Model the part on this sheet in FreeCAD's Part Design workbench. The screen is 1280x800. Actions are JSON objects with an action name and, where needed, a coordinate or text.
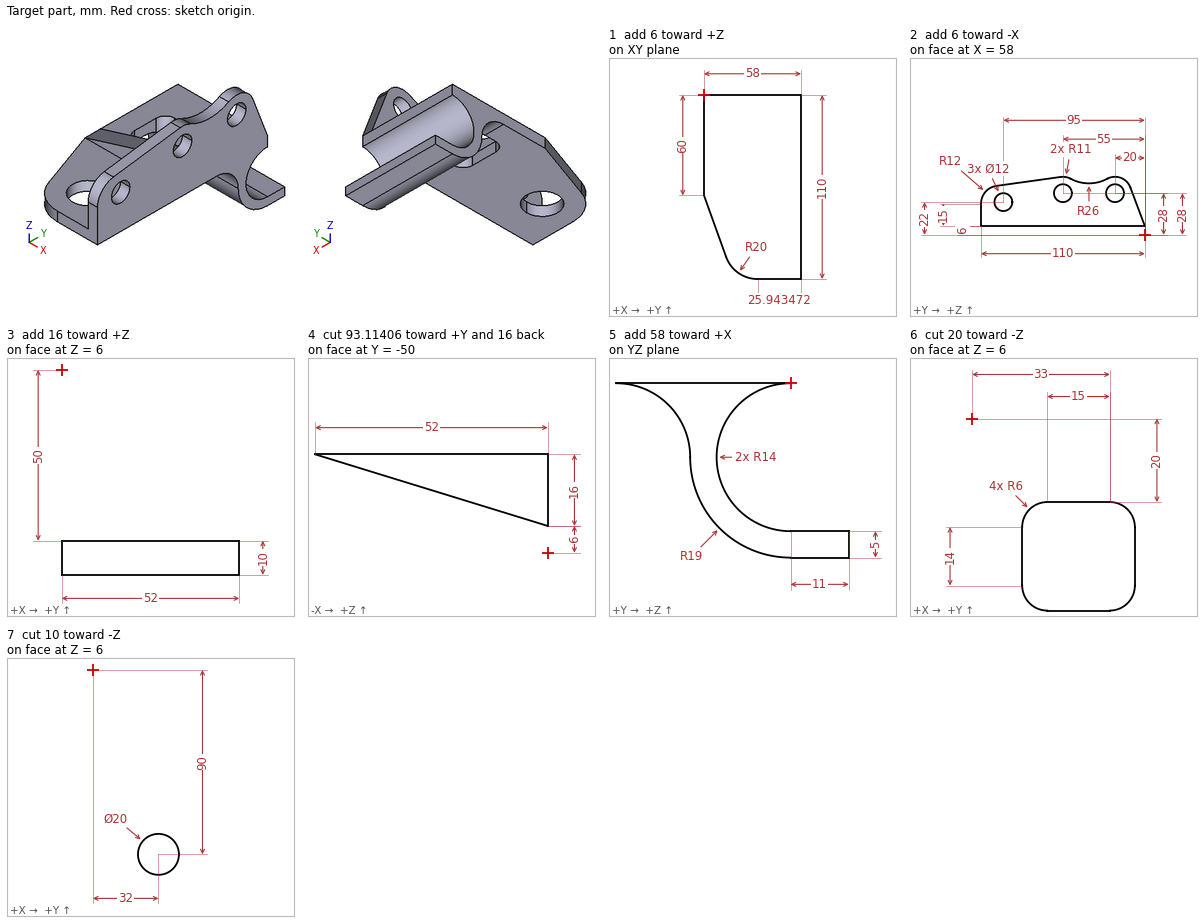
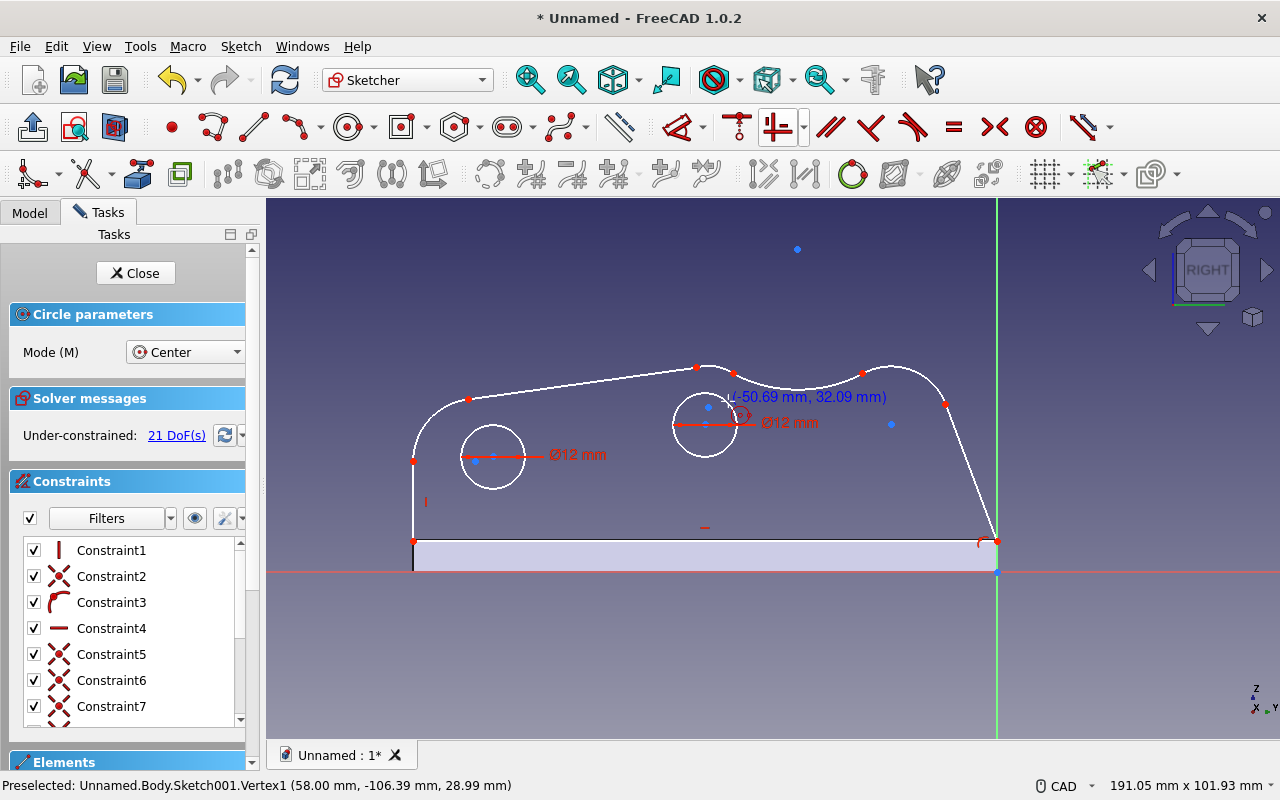
{"action": "left_click", "coordinate": [891, 424]}
{"action": "mouse_move", "coordinate": [913, 401]}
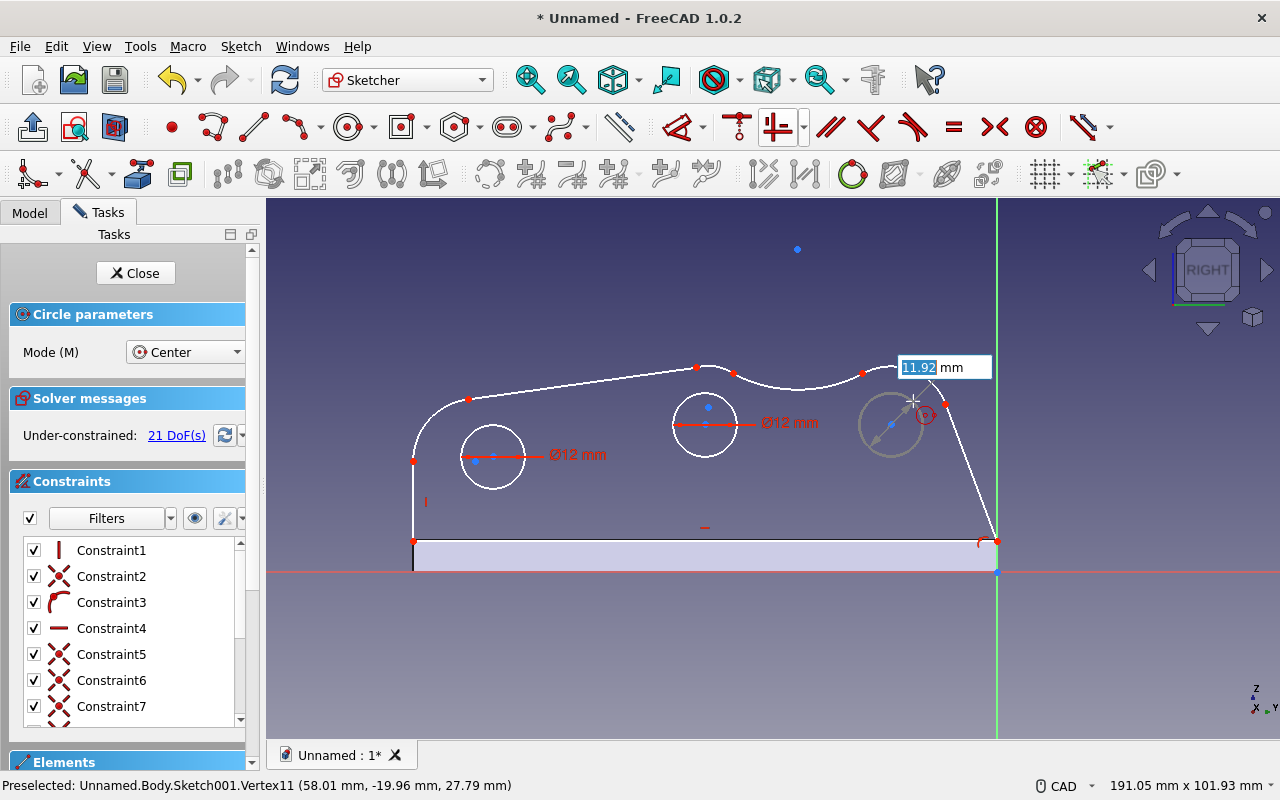
{"action": "type", "text": "12"}
{"action": "key", "text": "Return"}
{"action": "key", "text": "Escape"}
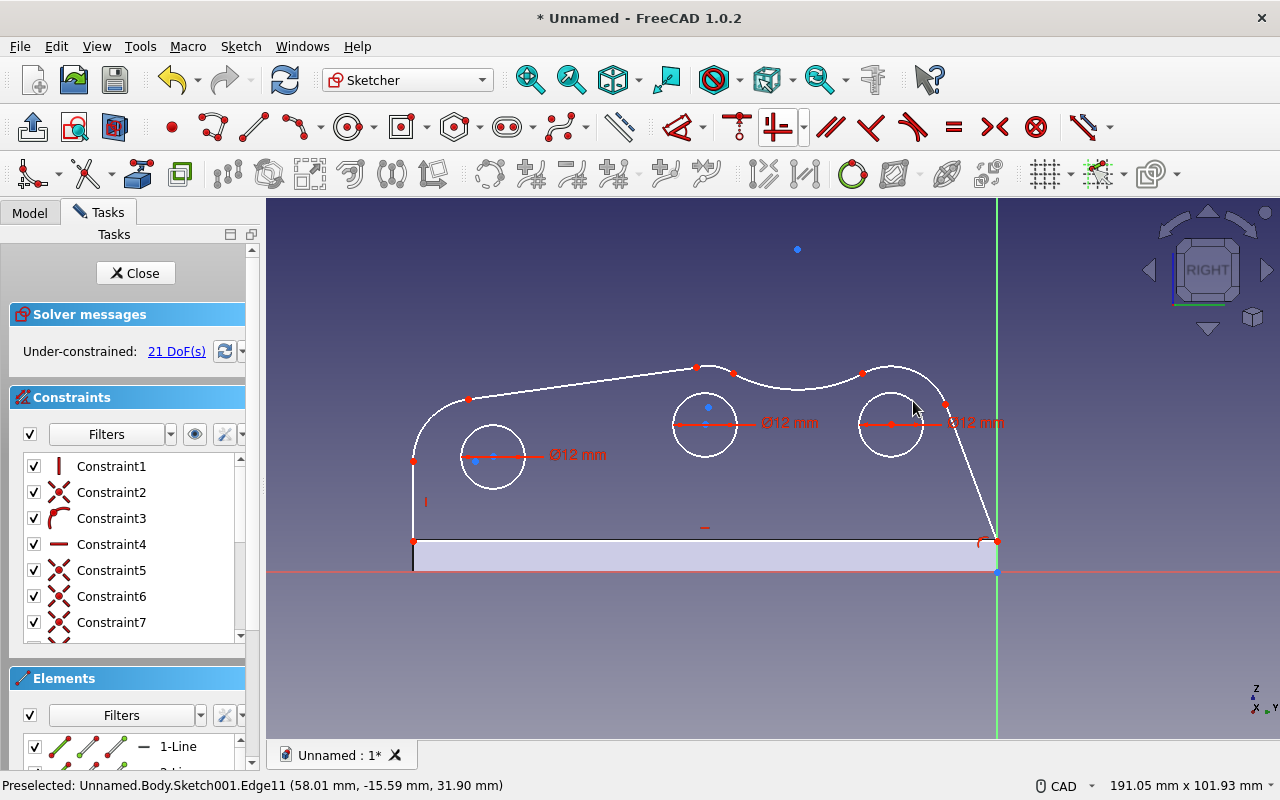
{"action": "left_click", "coordinate": [413, 486]}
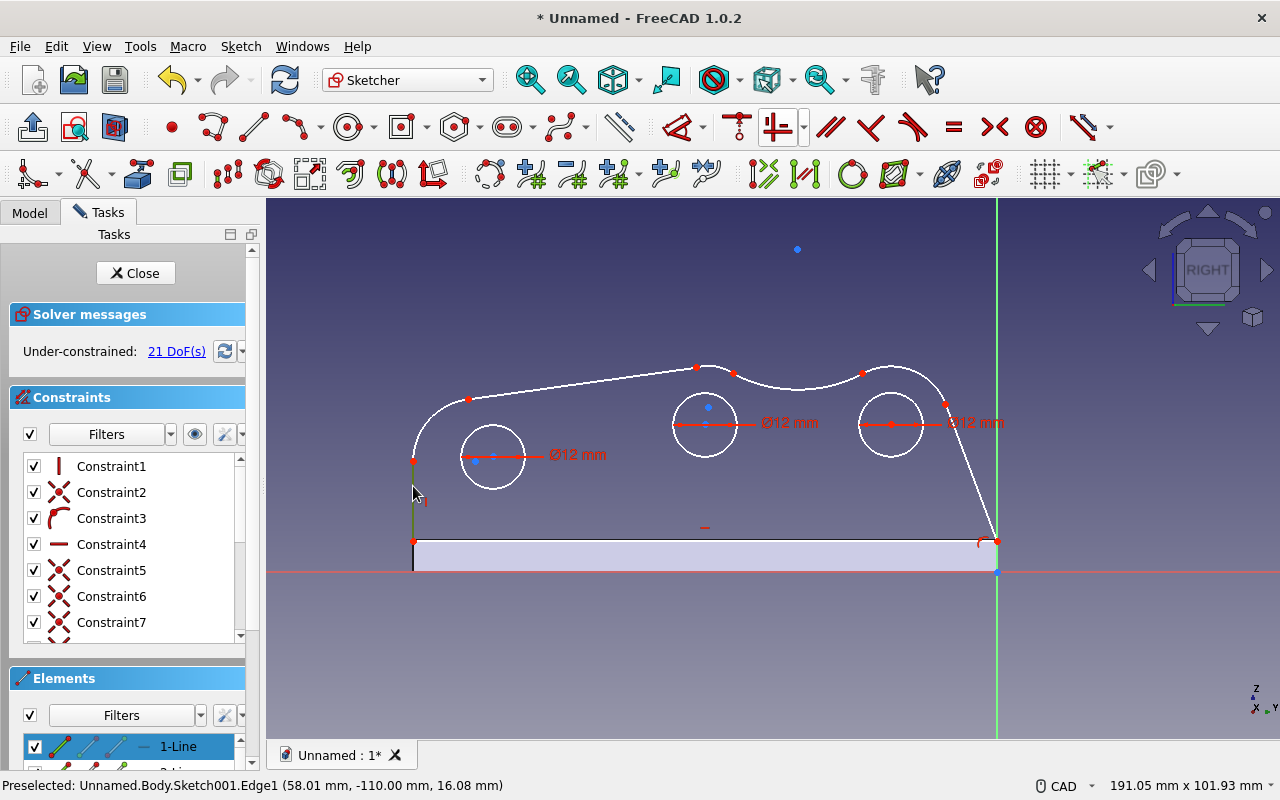
{"action": "left_click", "coordinate": [443, 408]}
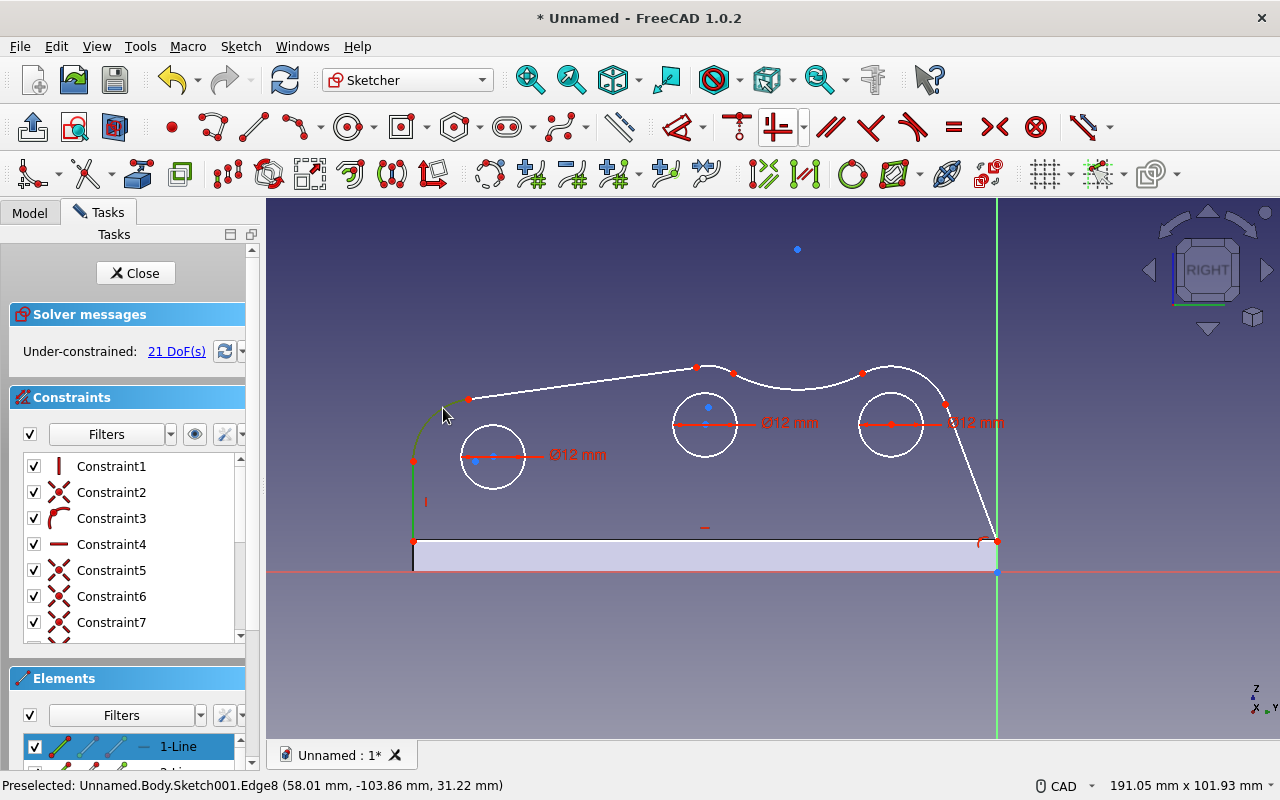
{"action": "key", "text": "t"}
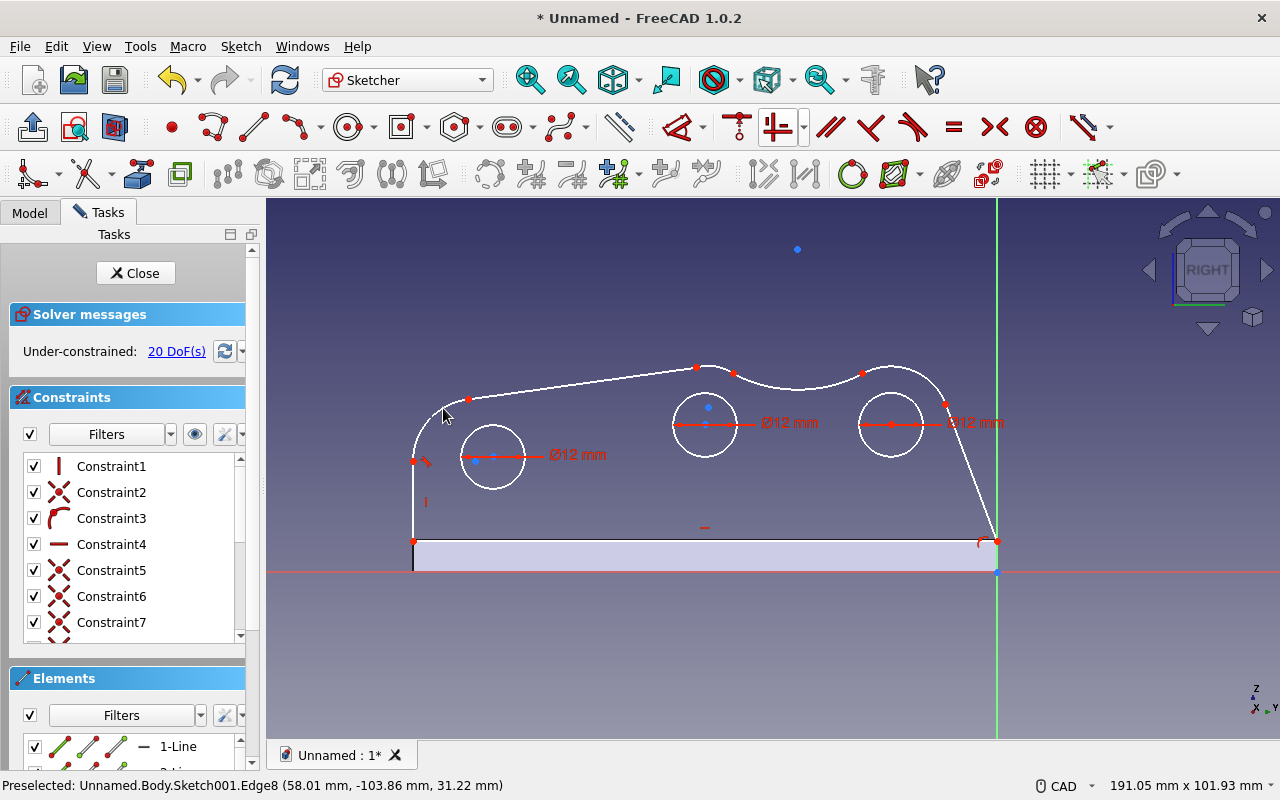
{"action": "left_click", "coordinate": [982, 500]}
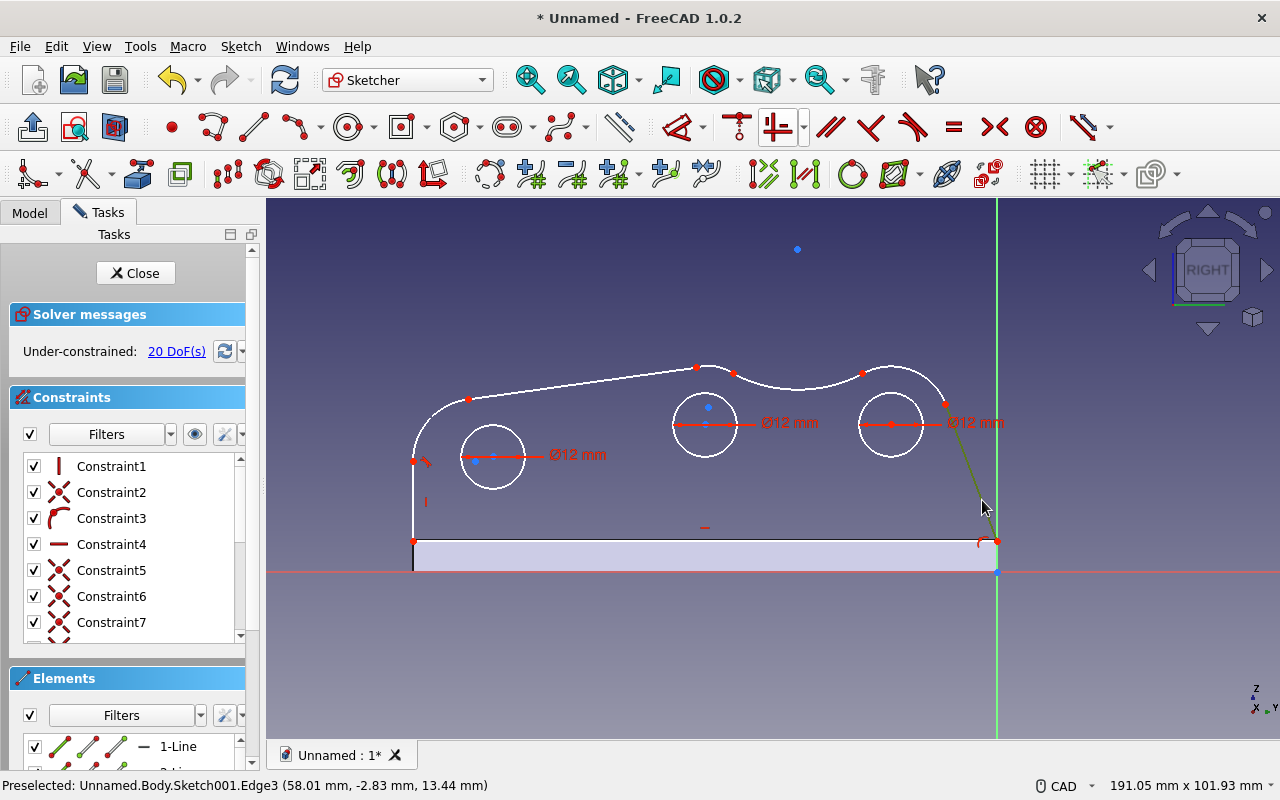
{"action": "left_click", "coordinate": [929, 380]}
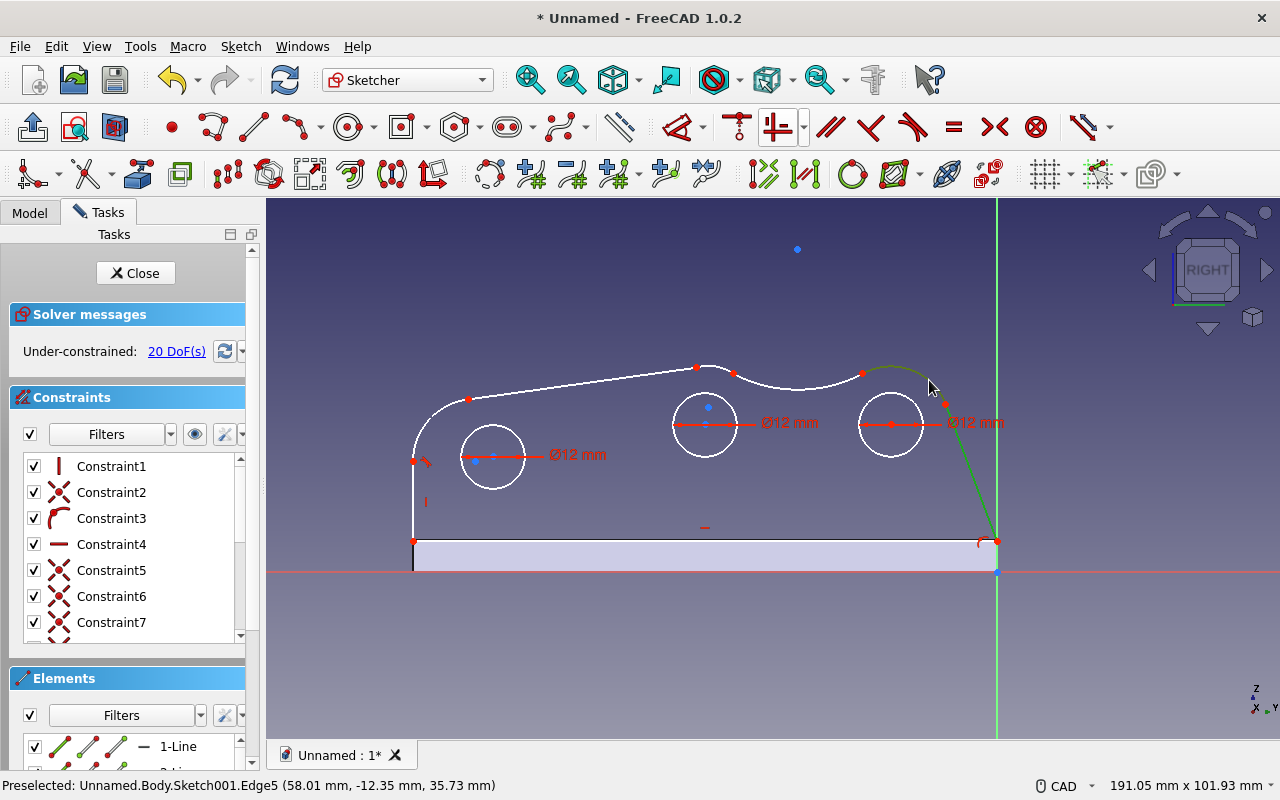
{"action": "left_click", "coordinate": [913, 128]}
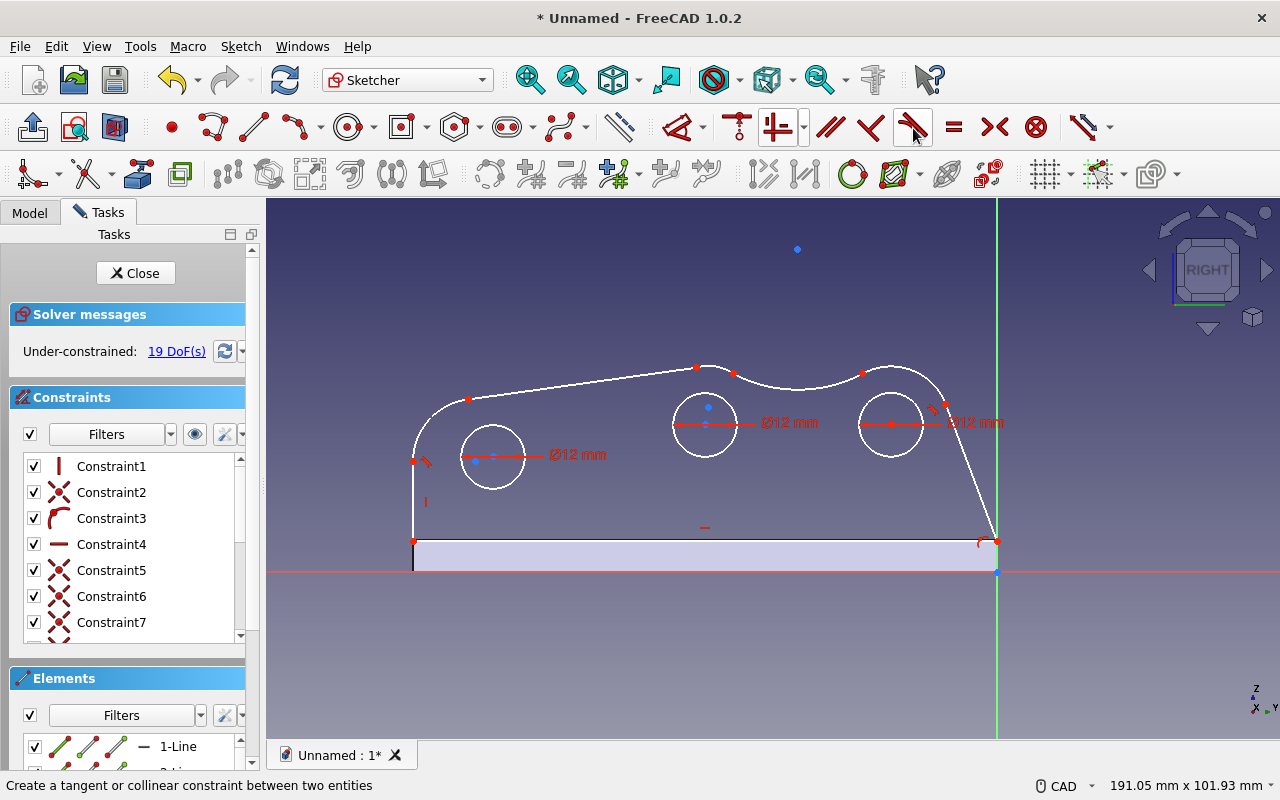
{"action": "left_click", "coordinate": [628, 377]}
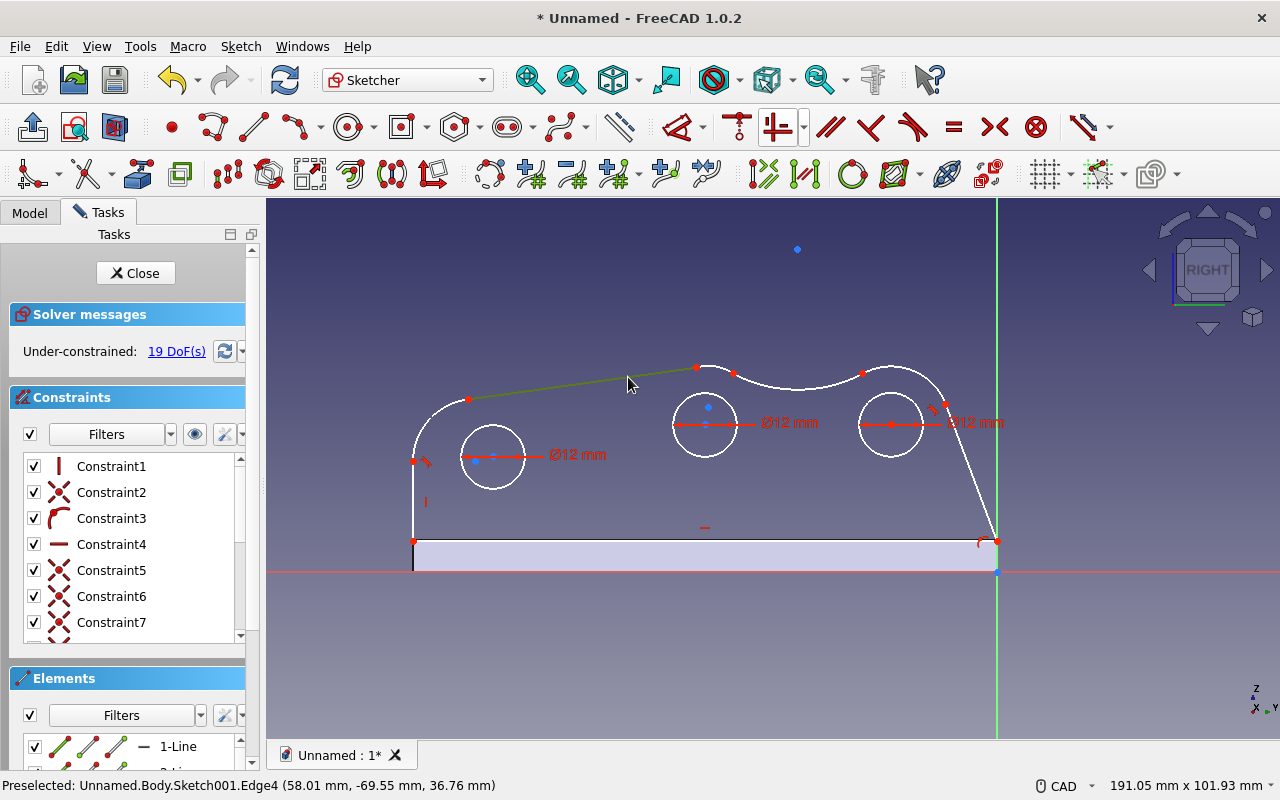
{"action": "left_click", "coordinate": [723, 368]}